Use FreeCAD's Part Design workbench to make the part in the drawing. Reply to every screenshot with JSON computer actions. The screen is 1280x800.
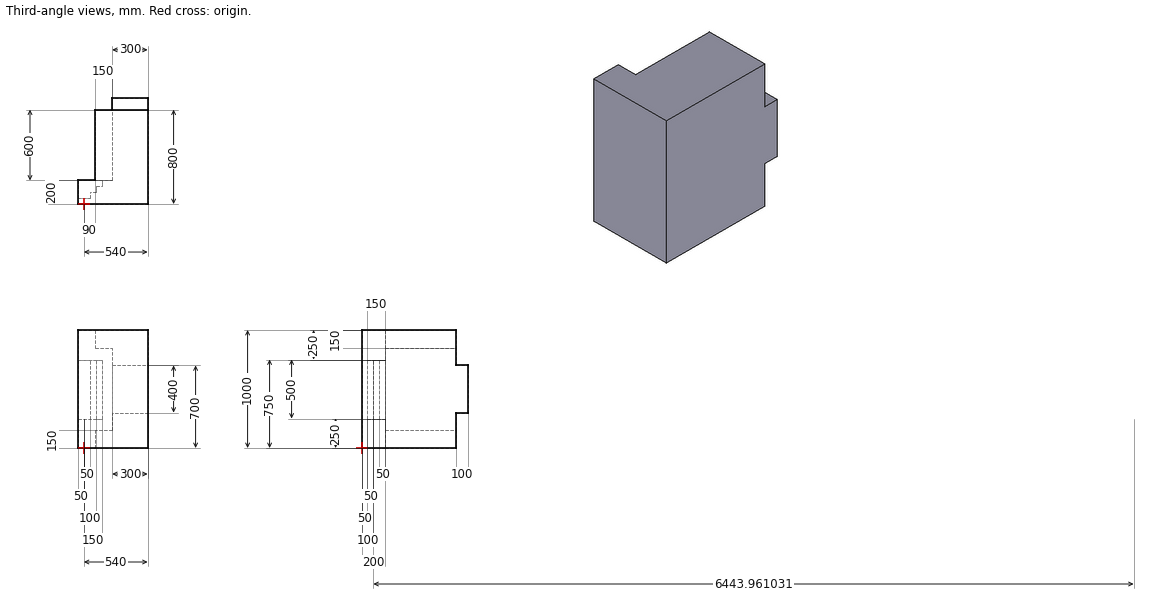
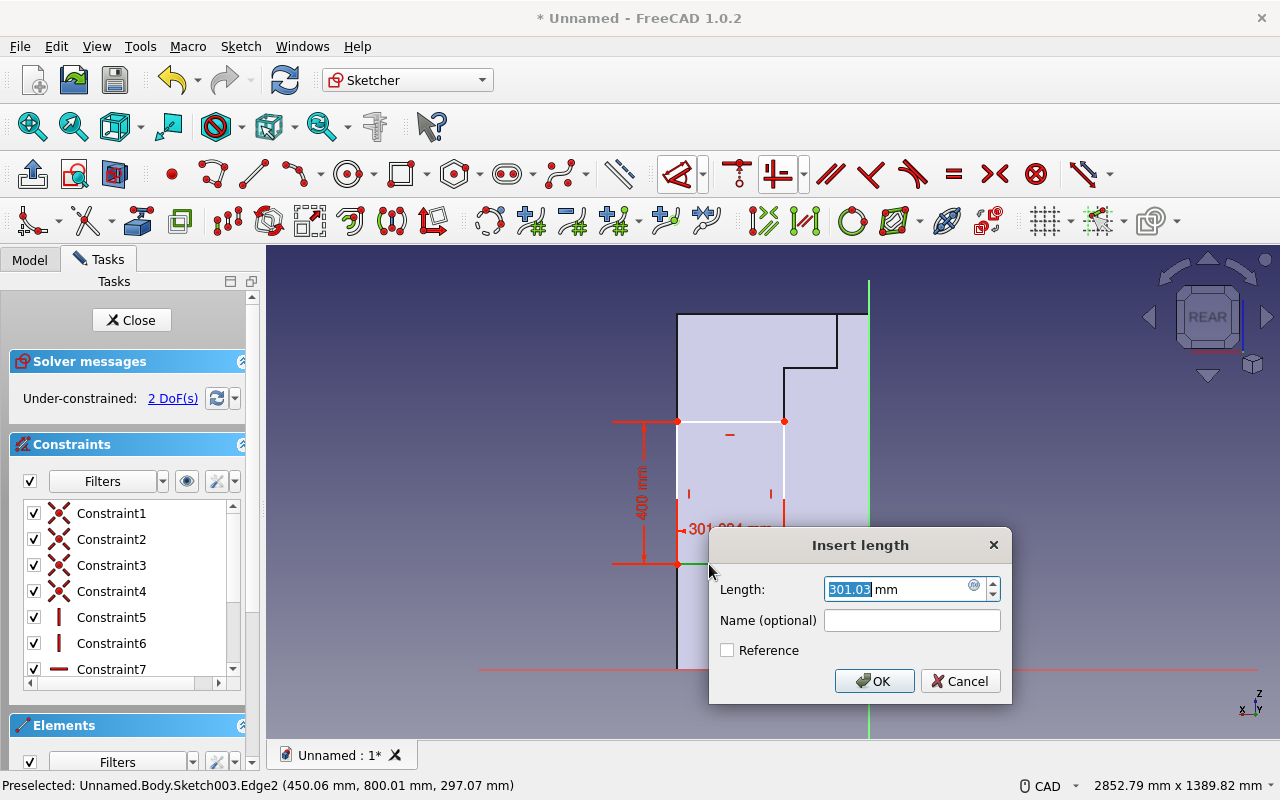
{"action": "type", "text": "300"}
{"action": "key", "text": "Return"}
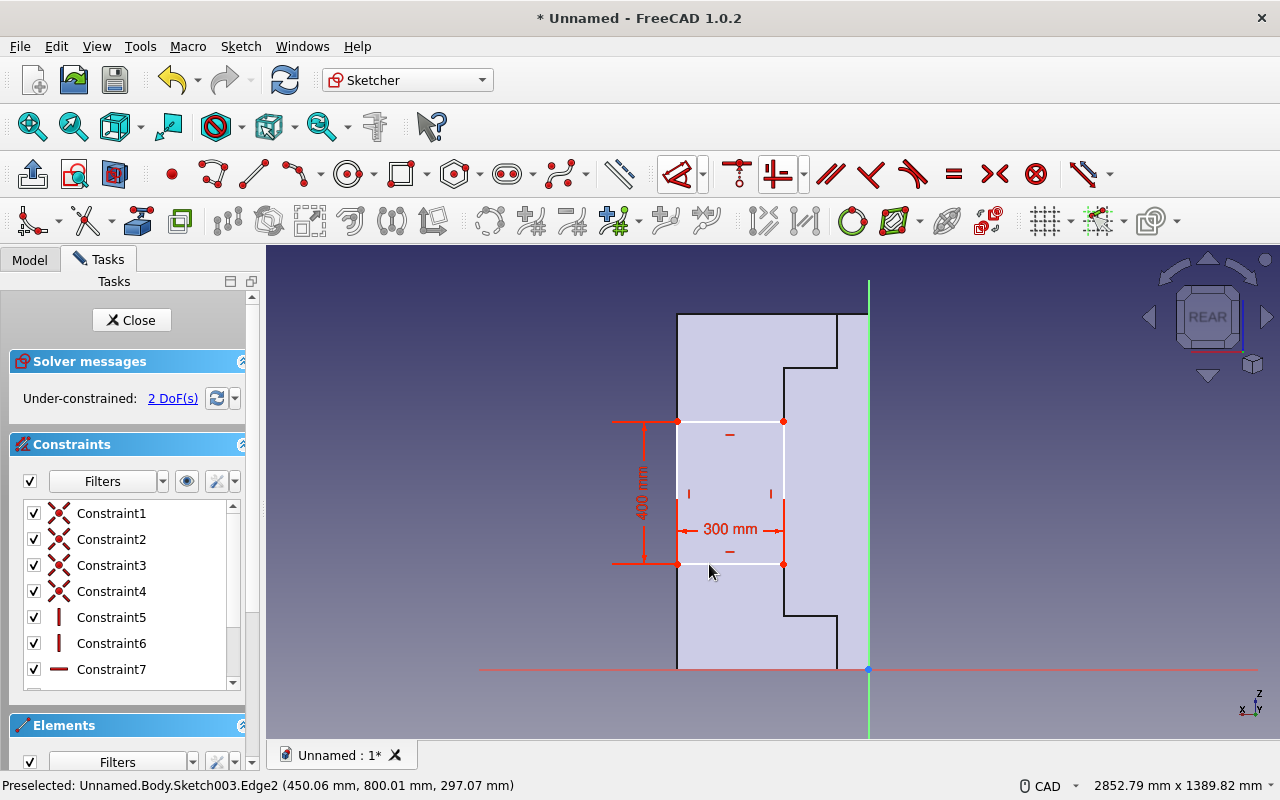
{"action": "left_click", "coordinate": [677, 422]}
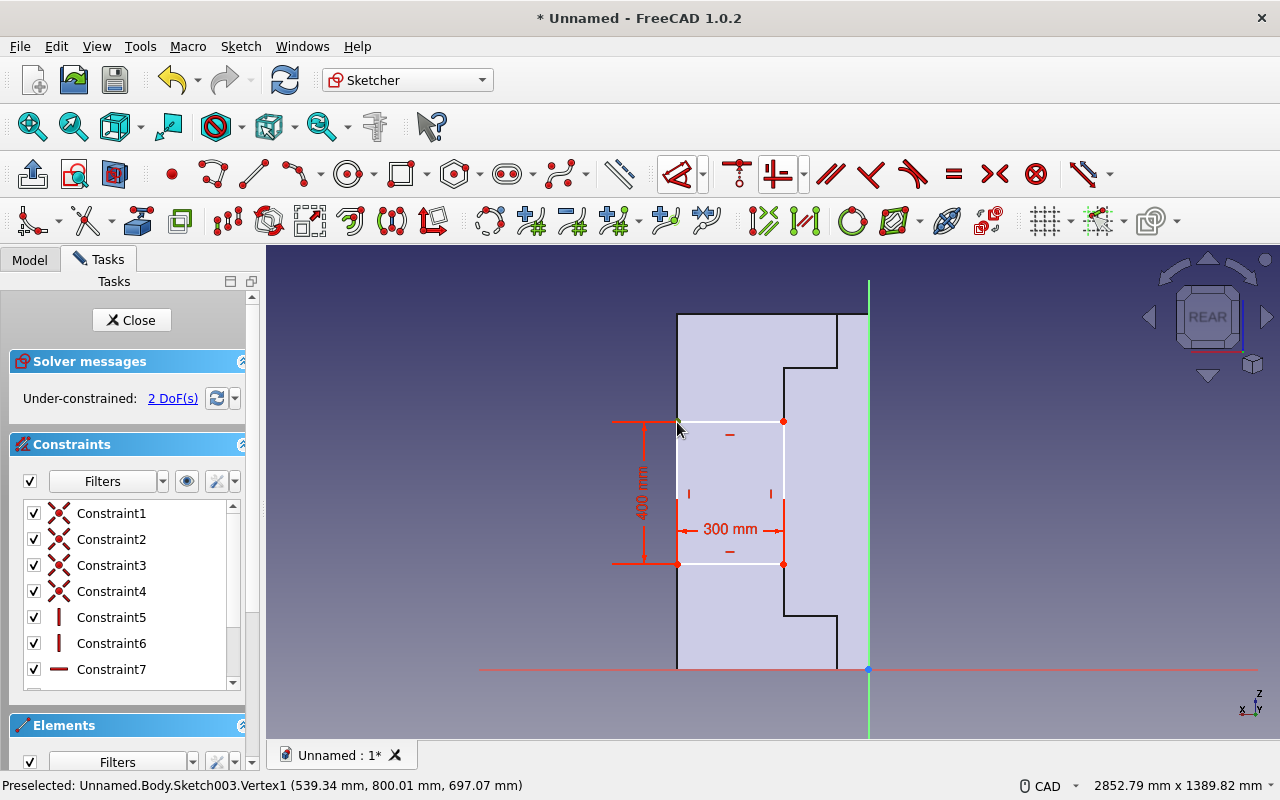
{"action": "left_click", "coordinate": [702, 174]}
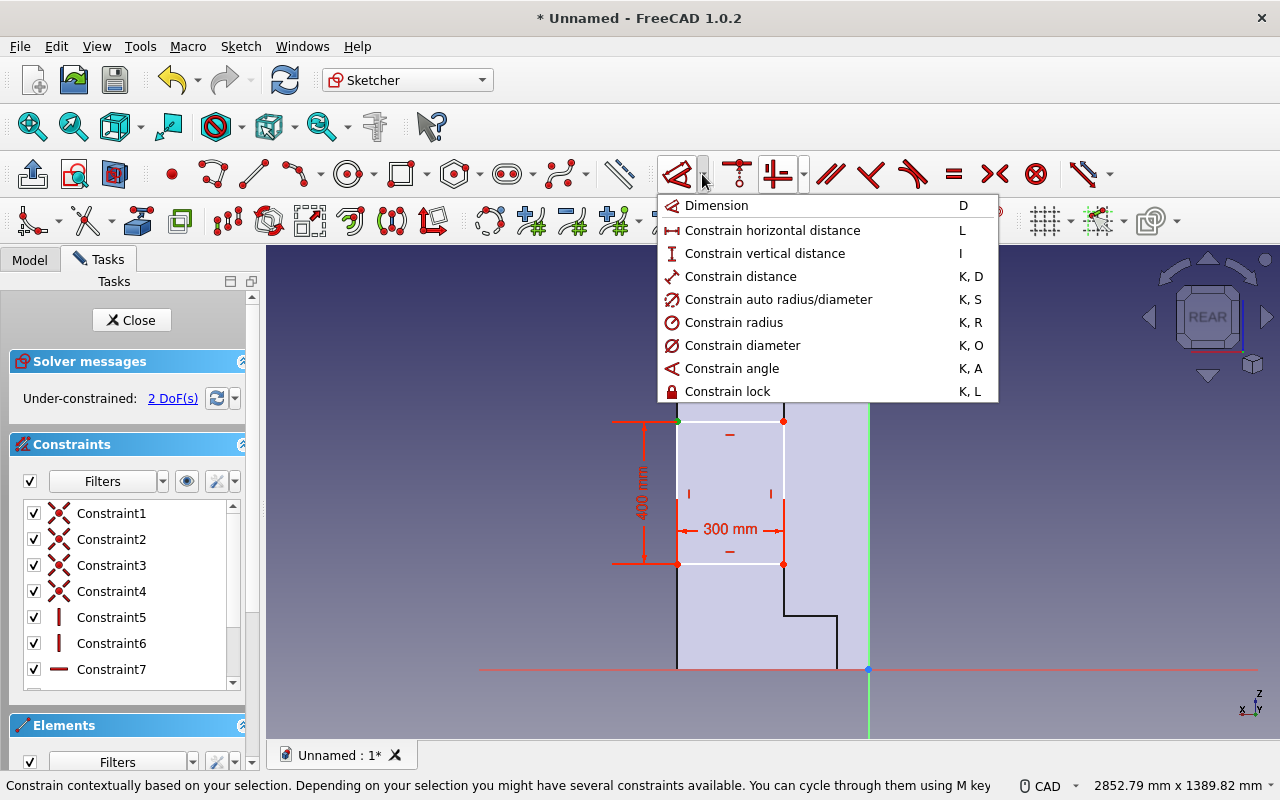
{"action": "left_click", "coordinate": [828, 230]}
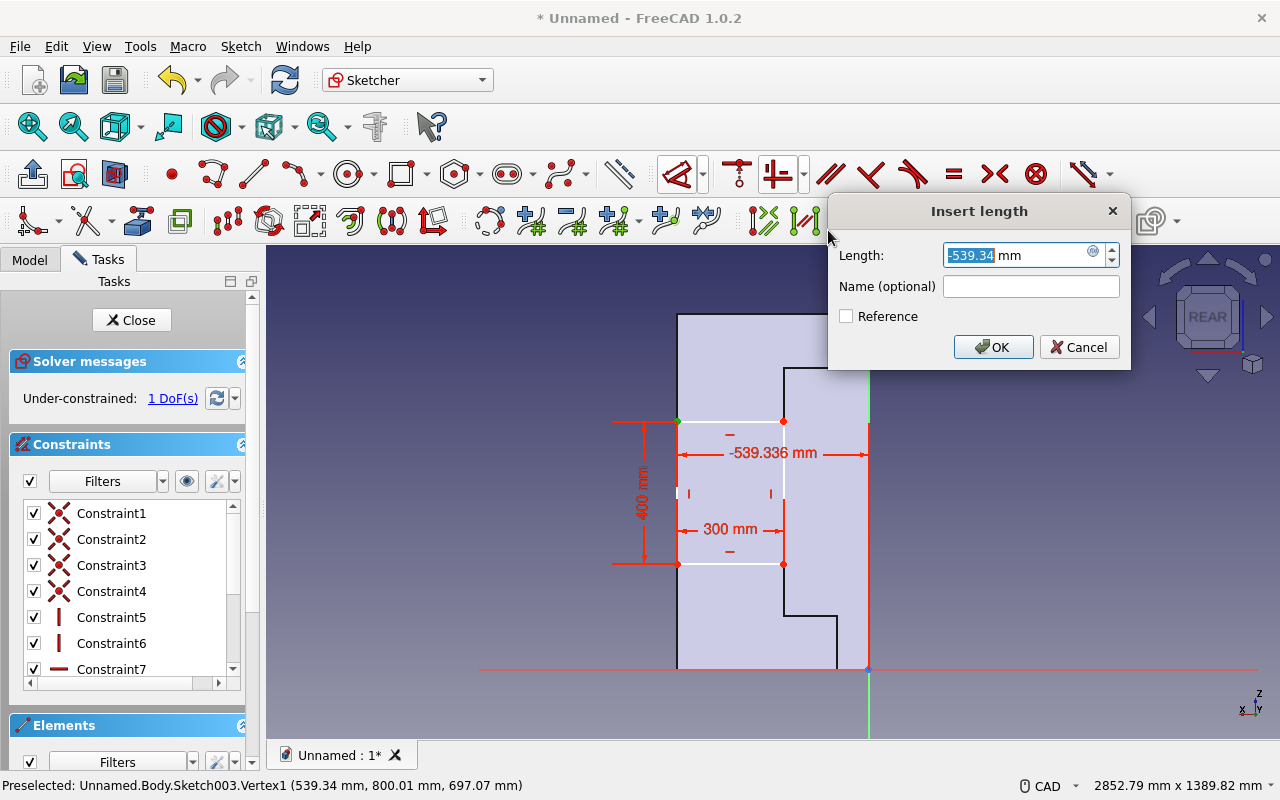
{"action": "type", "text": "-540"}
{"action": "key", "text": "Return"}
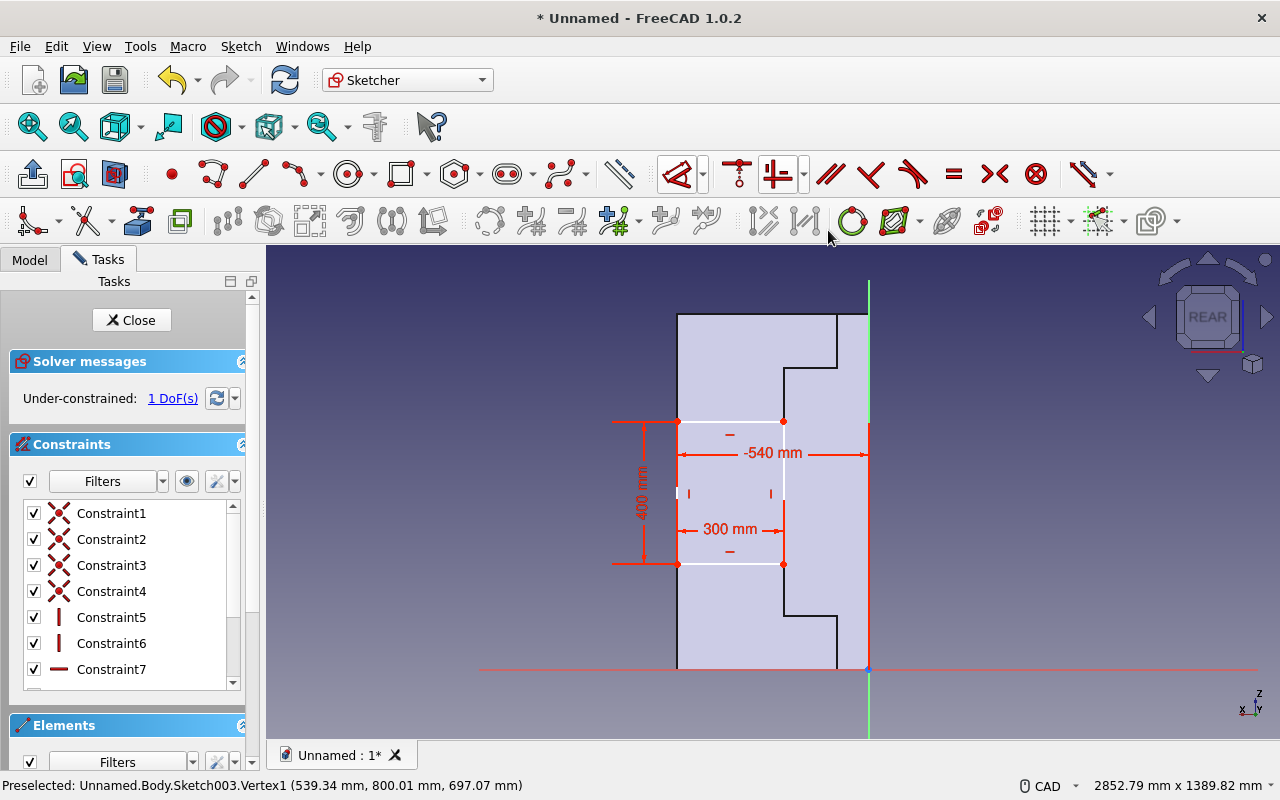
{"action": "left_click", "coordinate": [677, 422]}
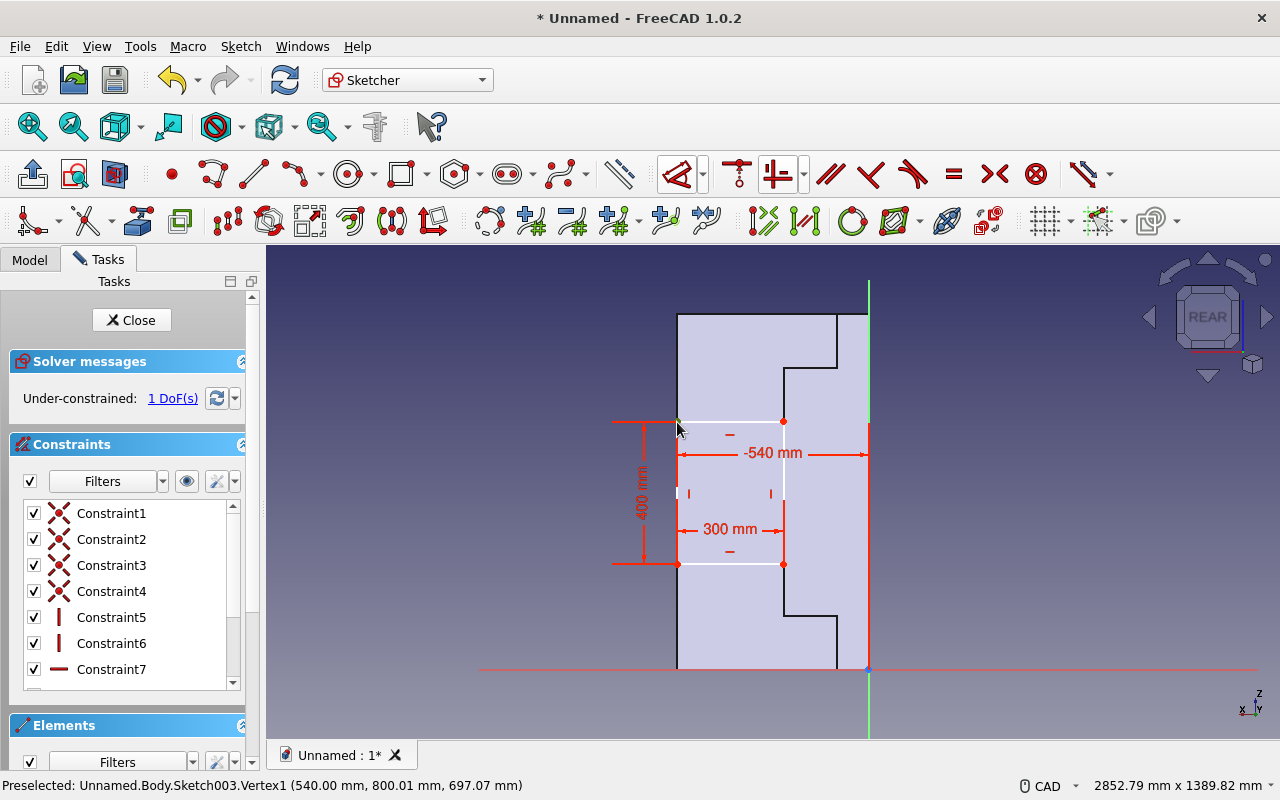
{"action": "left_click", "coordinate": [702, 174]}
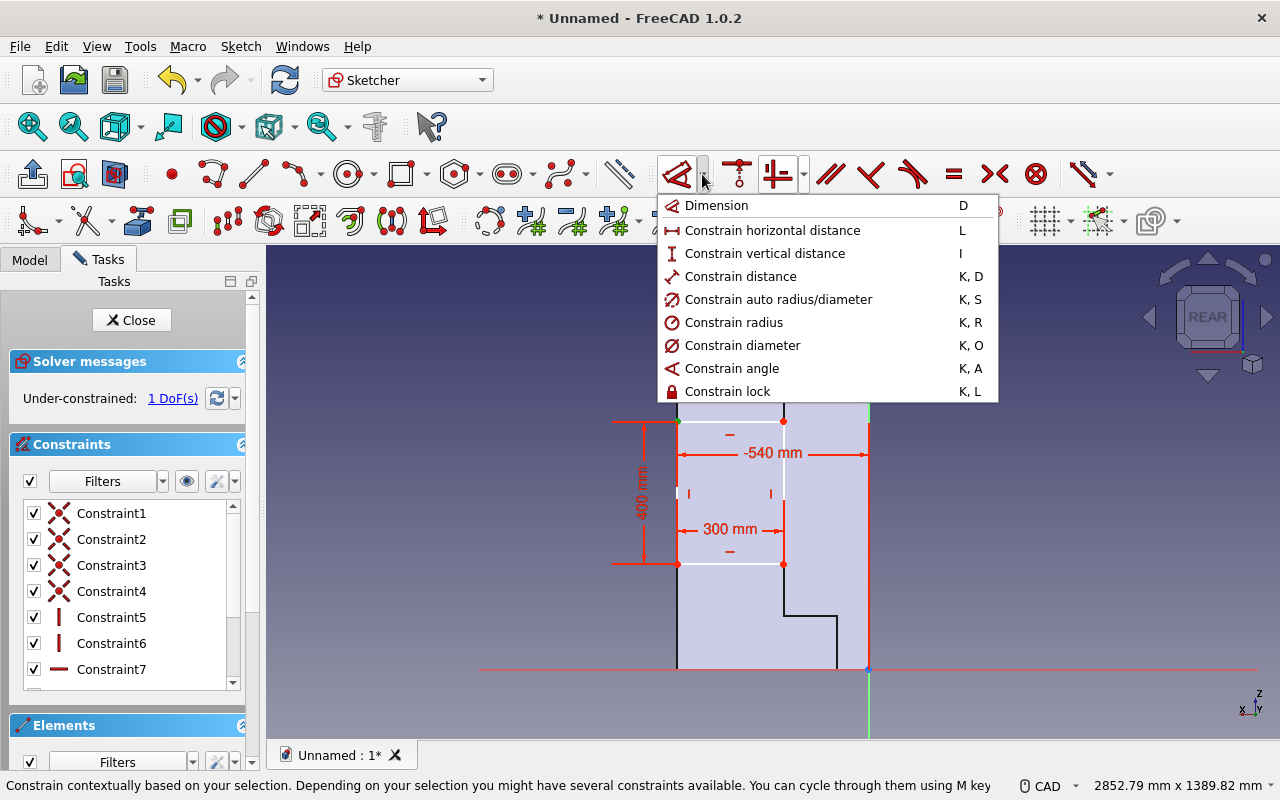
{"action": "left_click", "coordinate": [828, 254]}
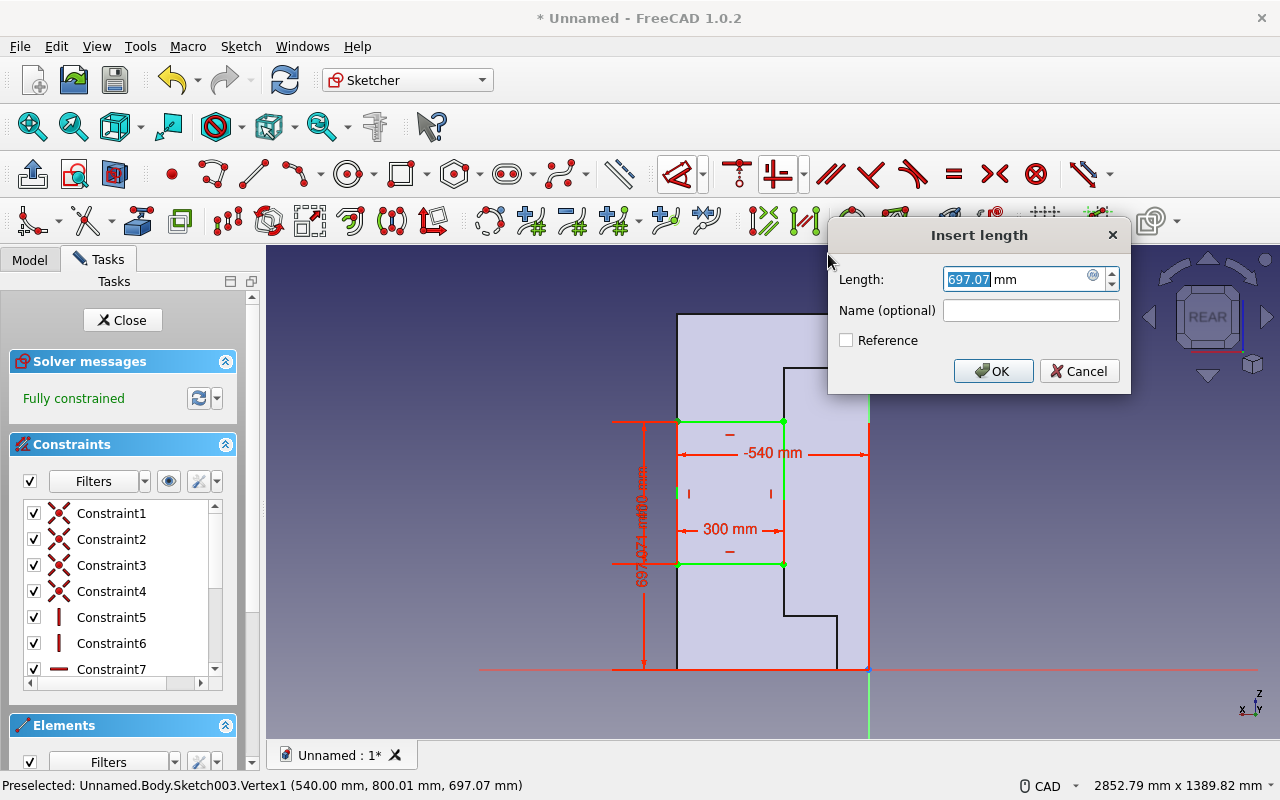
{"action": "type", "text": "700"}
{"action": "key", "text": "Return"}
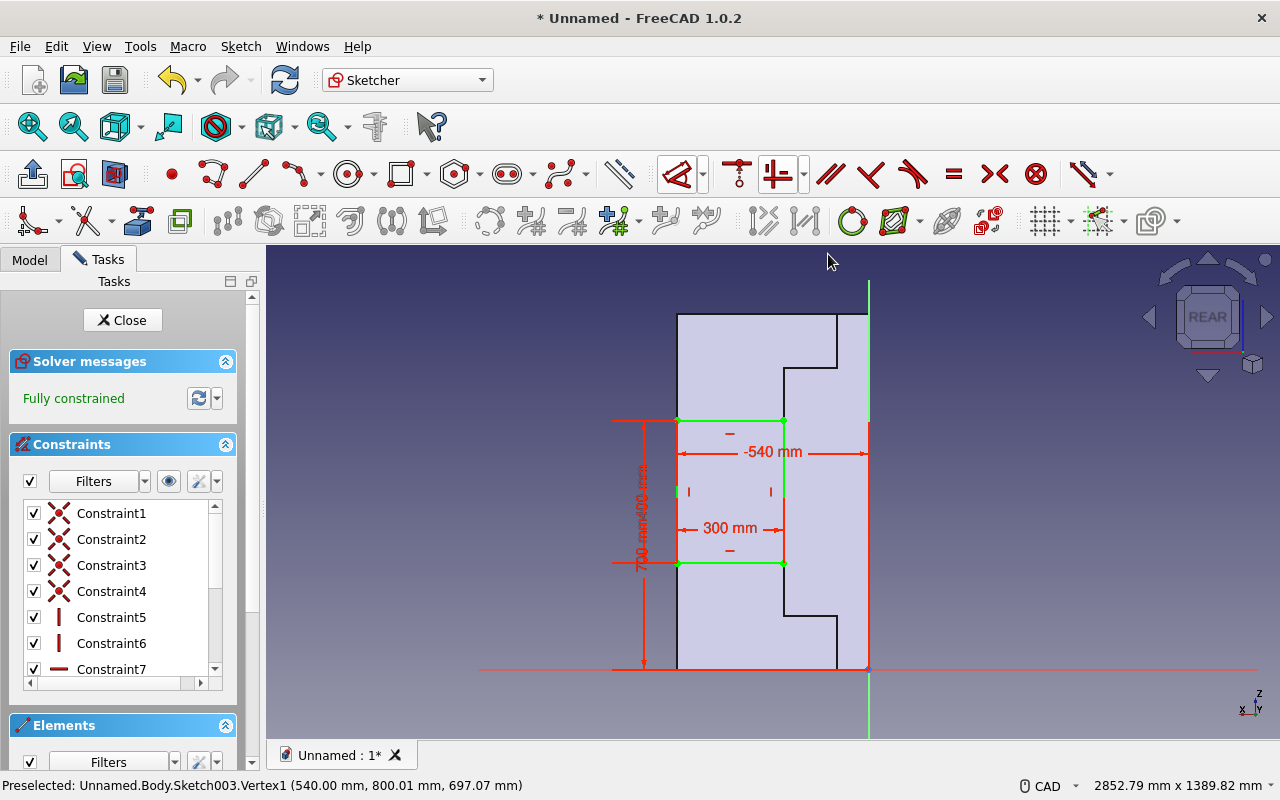
{"action": "left_click", "coordinate": [123, 320]}